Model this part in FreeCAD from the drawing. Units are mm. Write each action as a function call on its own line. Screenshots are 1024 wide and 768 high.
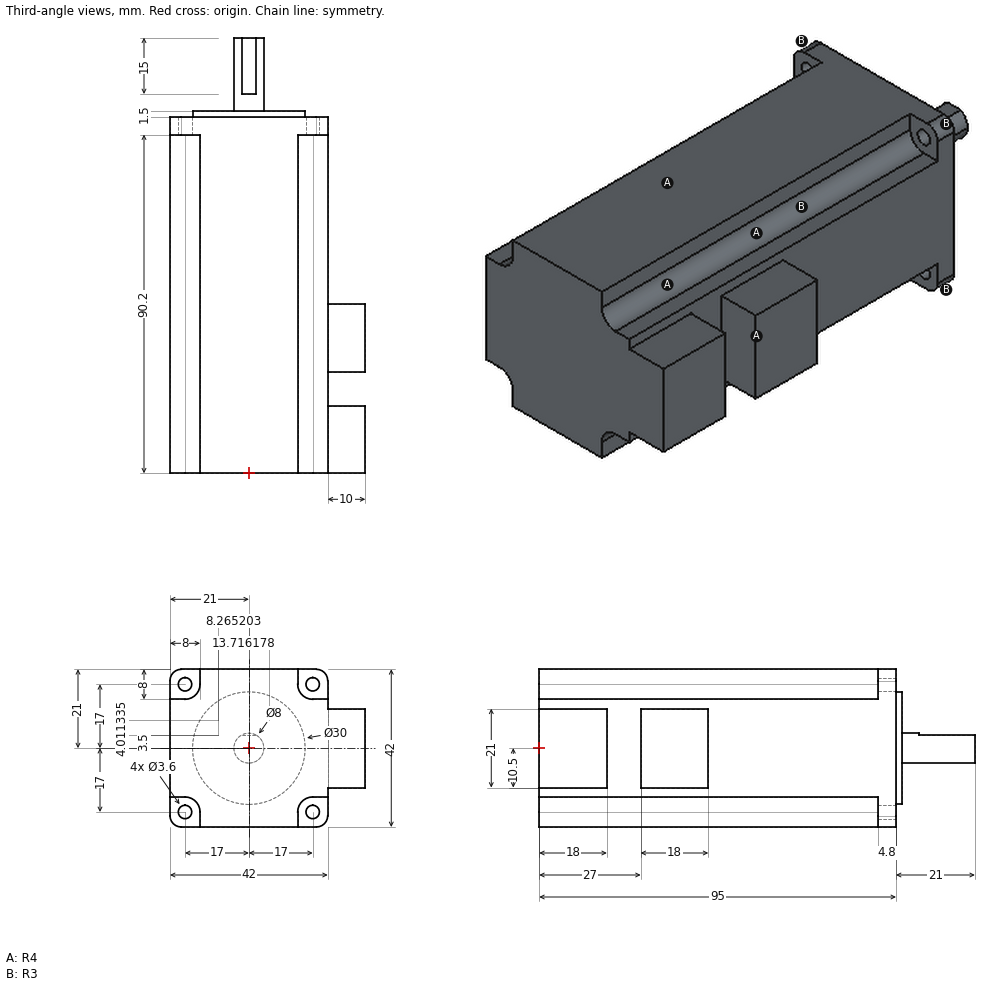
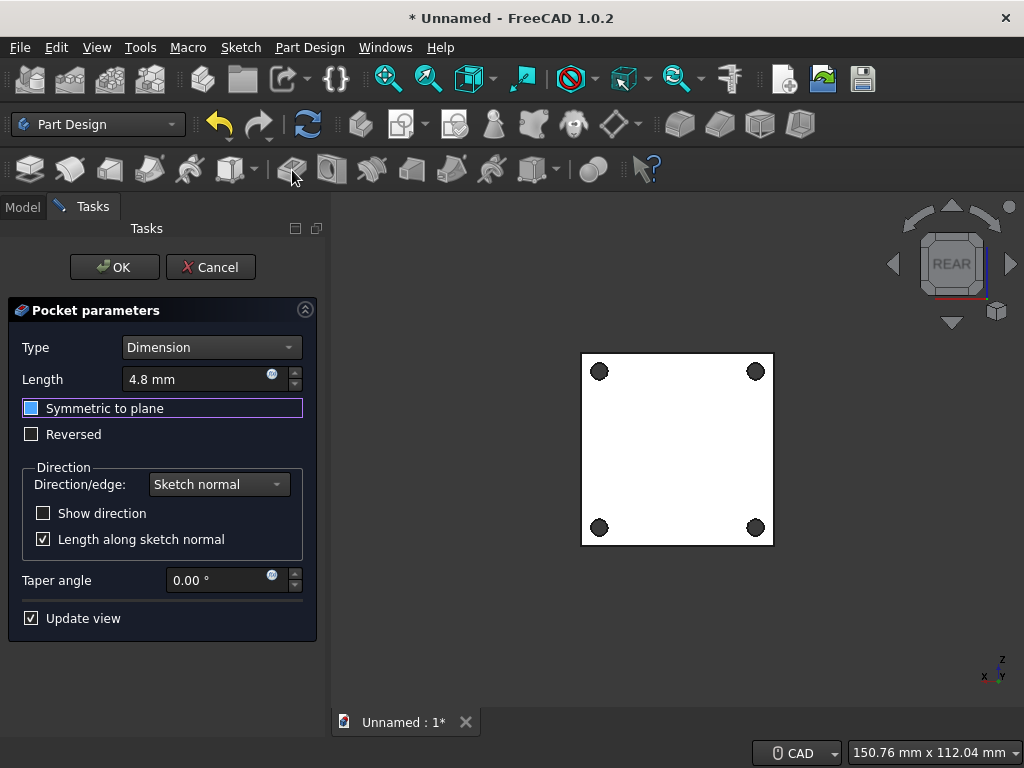
click(115, 267)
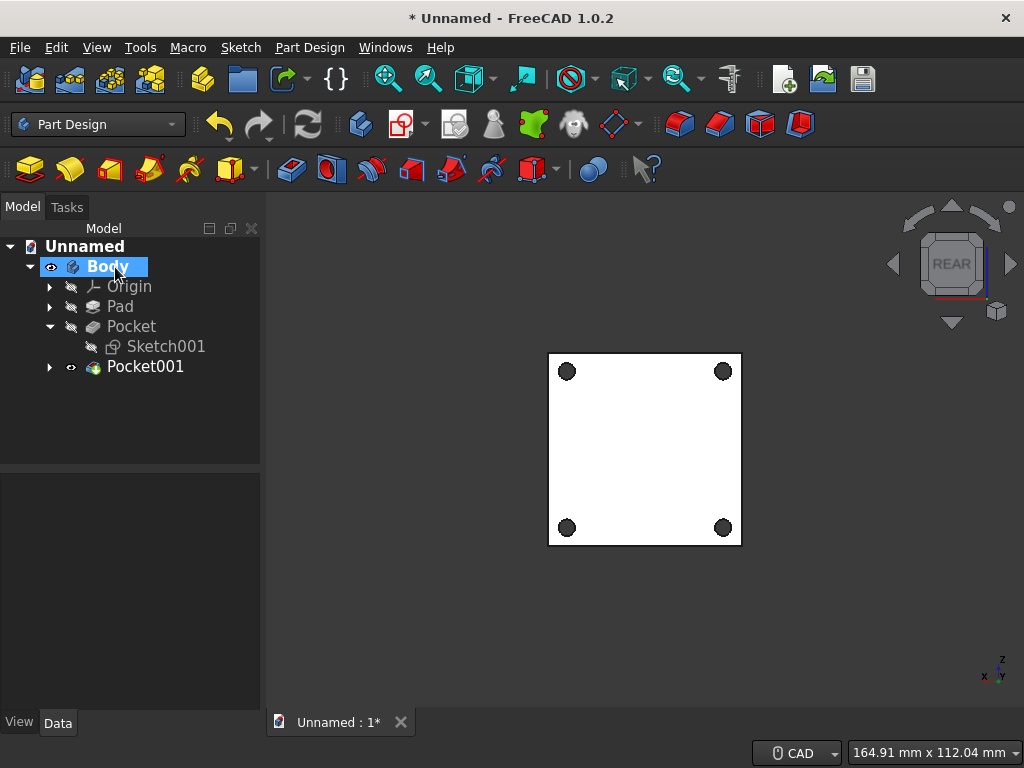
key(v)
key(f)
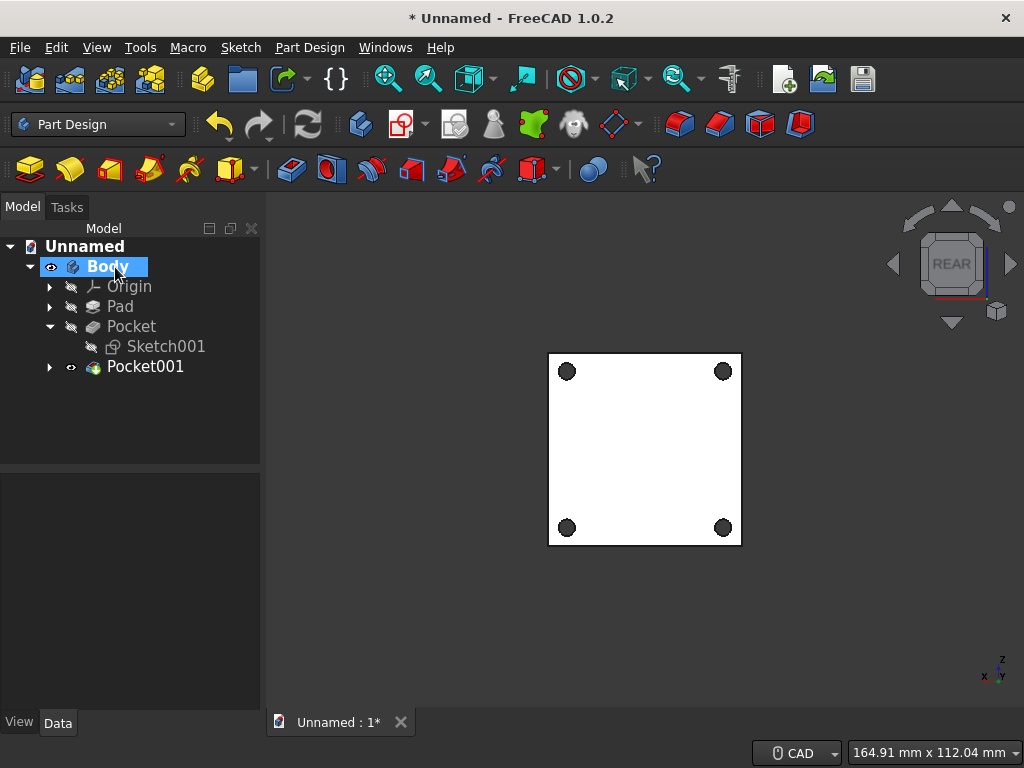
key(0)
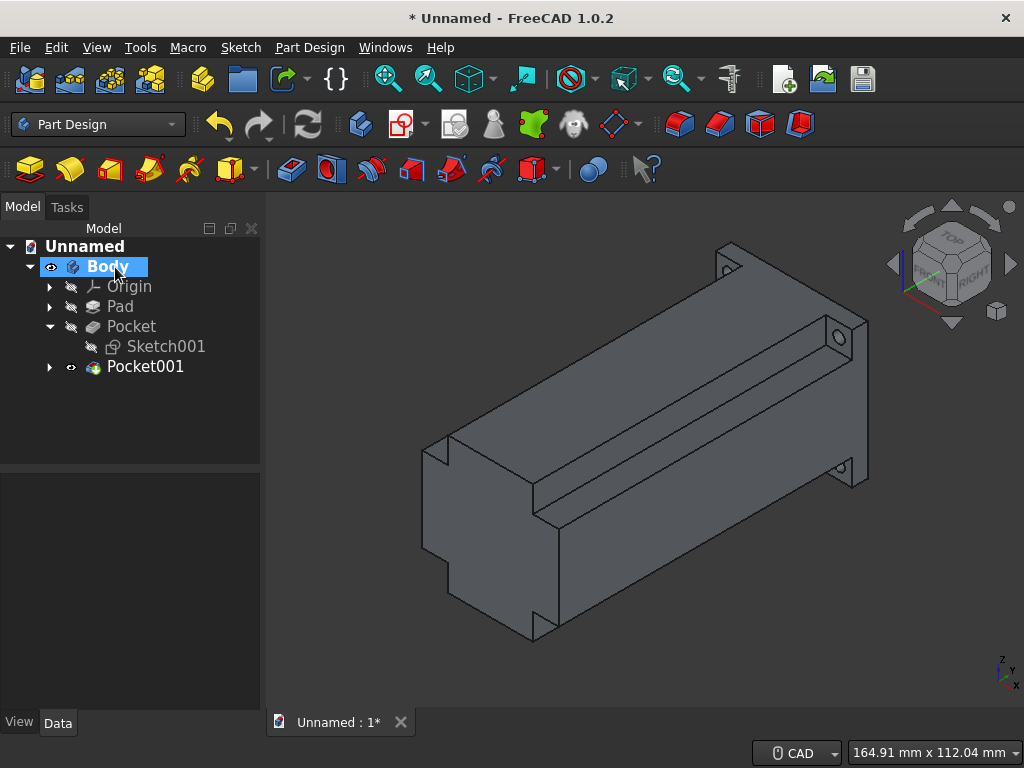
key(2)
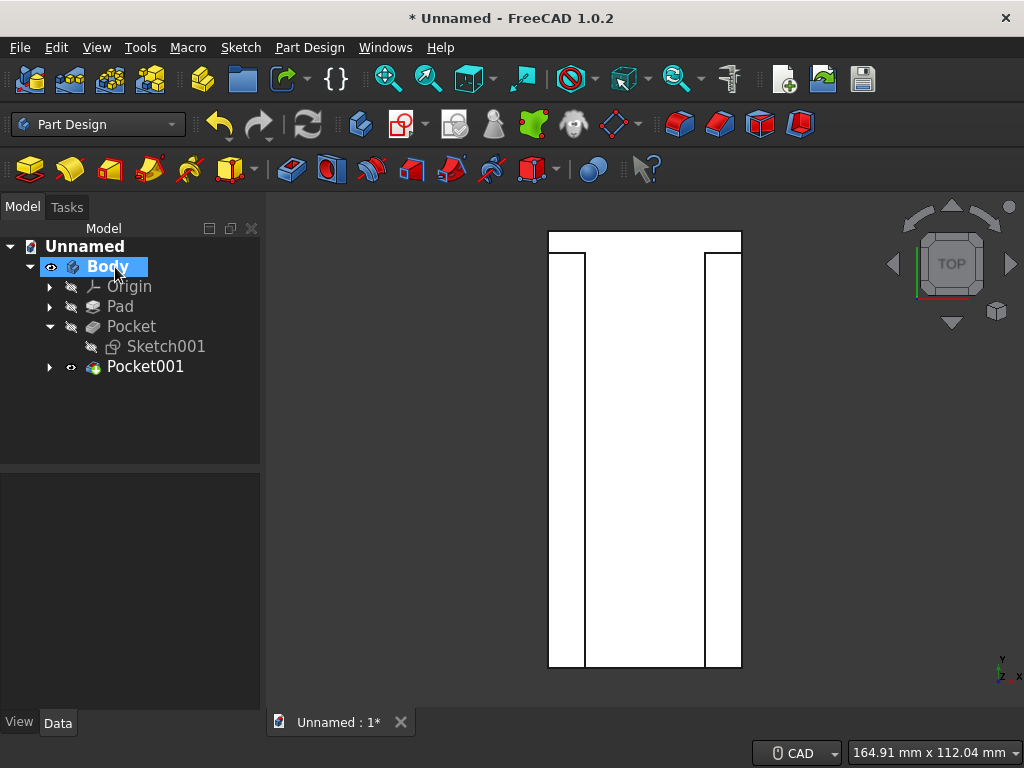
key(1)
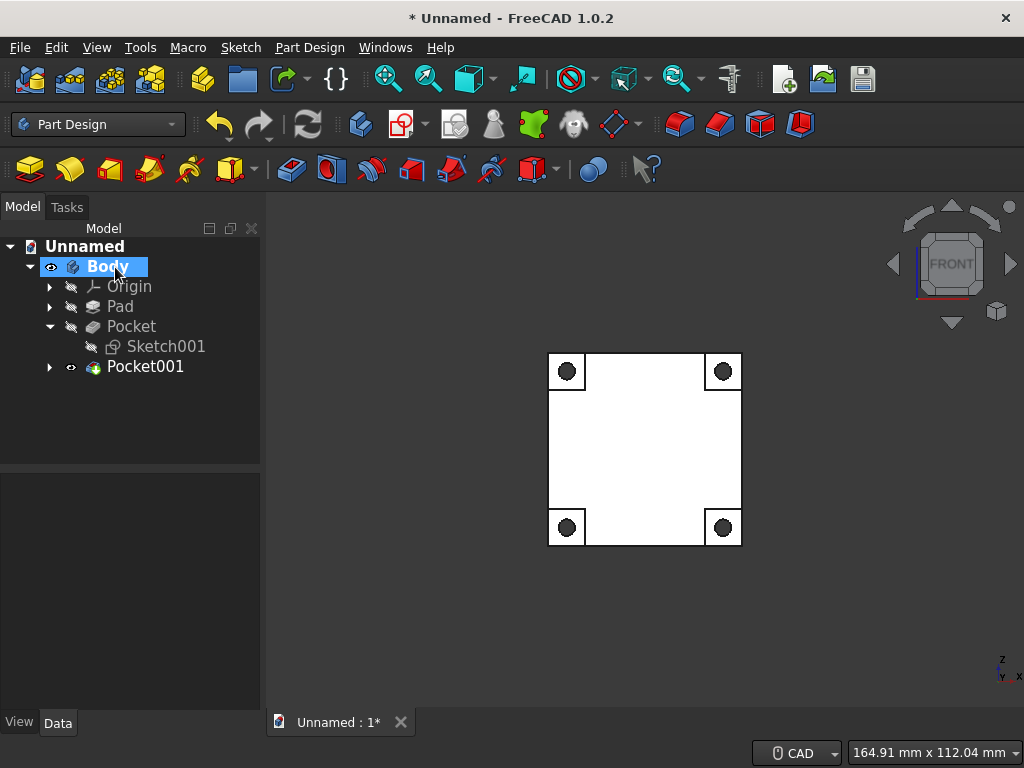
click(390, 80)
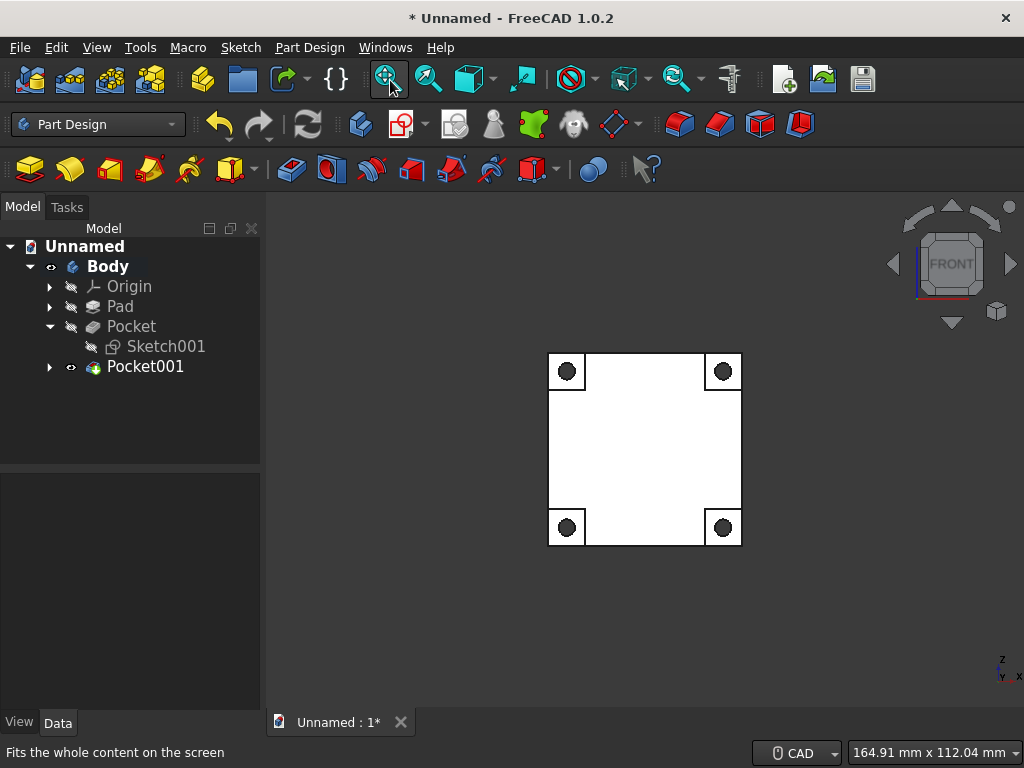
key(3)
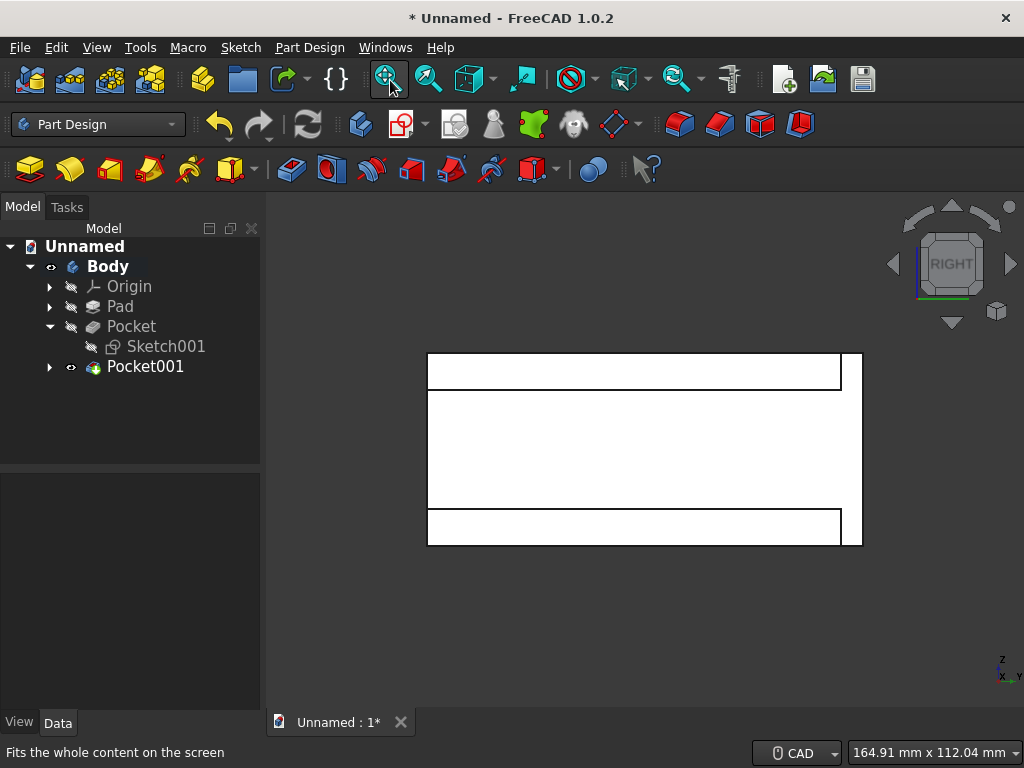
key(5)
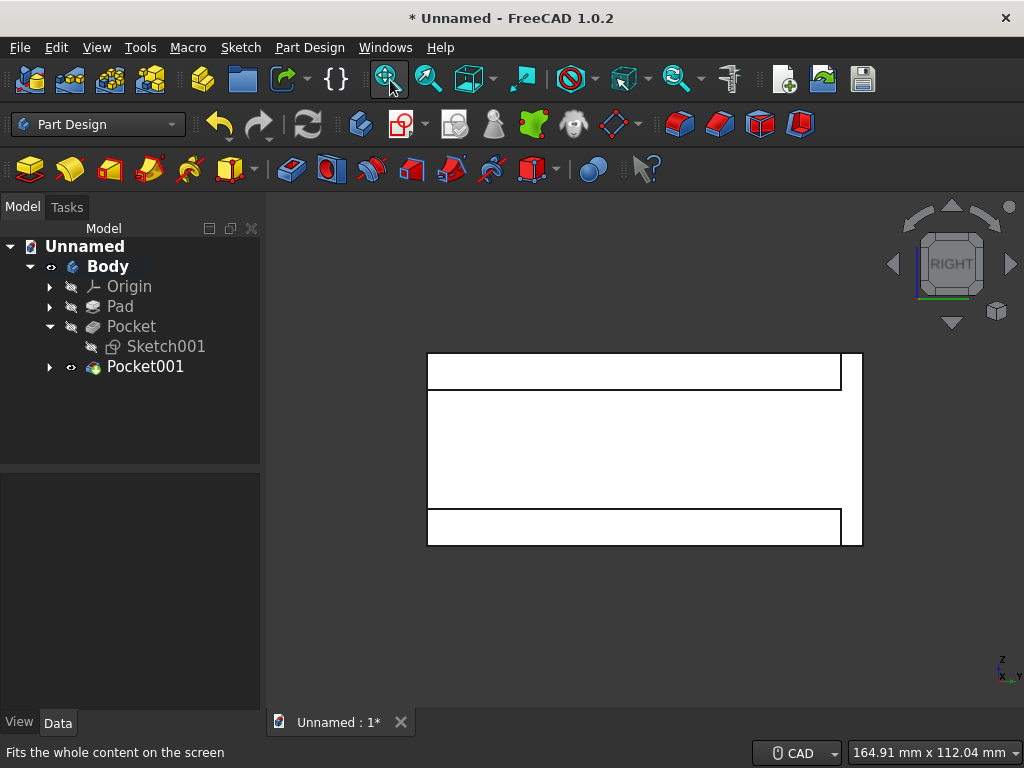
key(4)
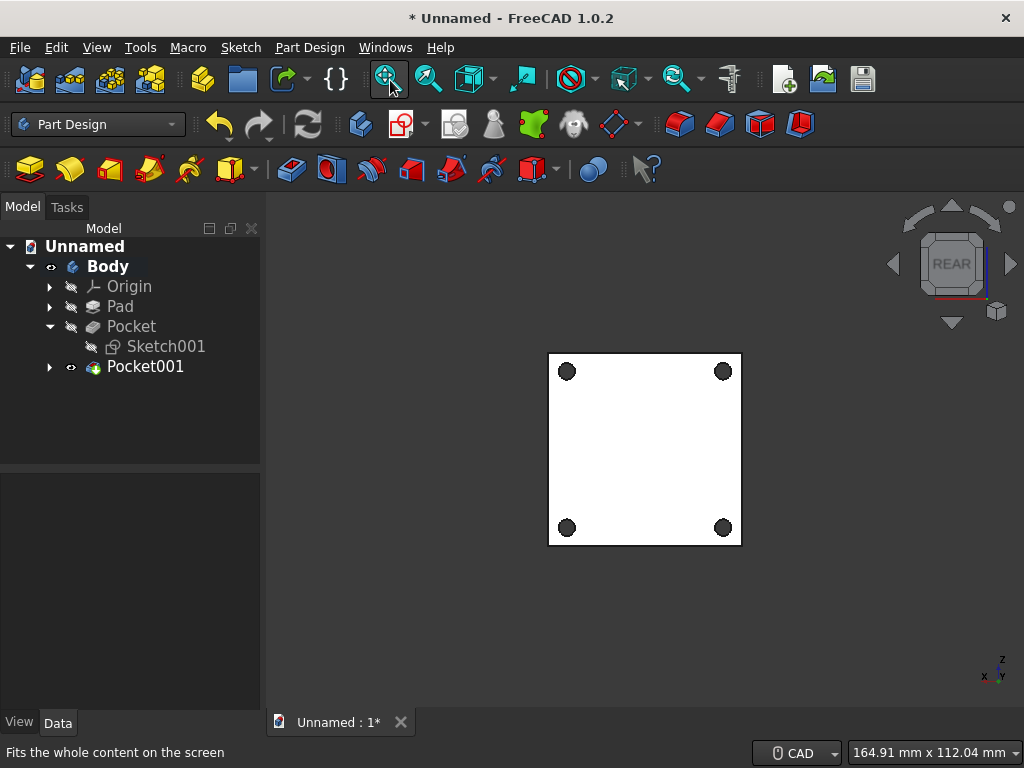
click(390, 80)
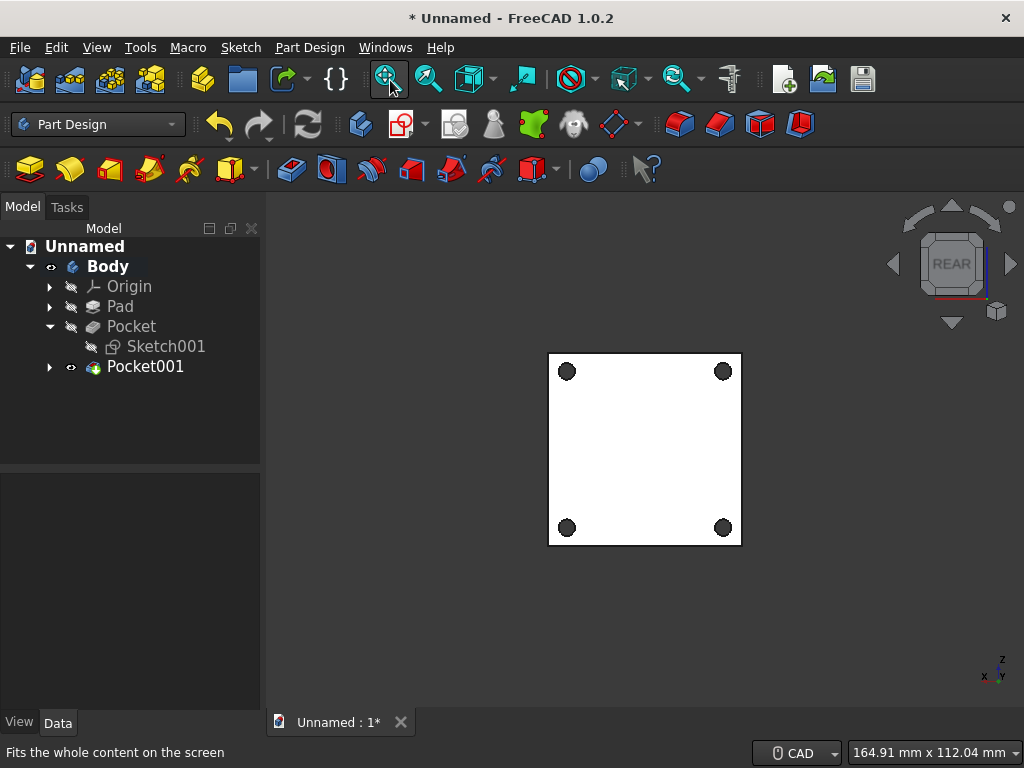
key(6)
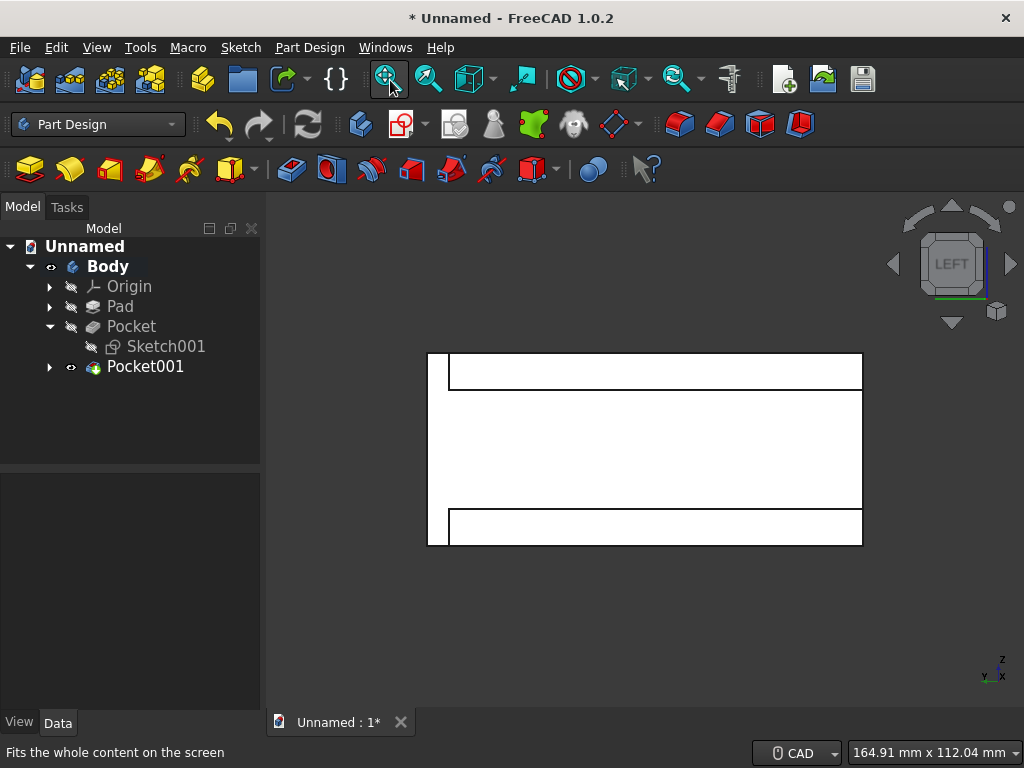
key(v)
key(3)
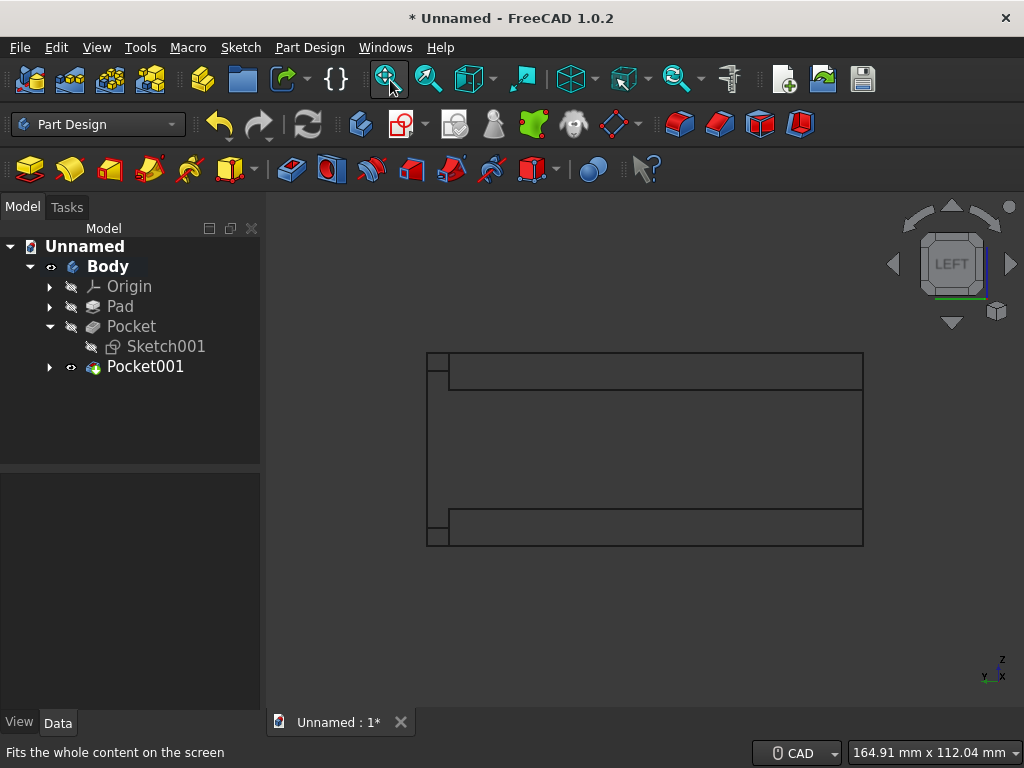
key(0)